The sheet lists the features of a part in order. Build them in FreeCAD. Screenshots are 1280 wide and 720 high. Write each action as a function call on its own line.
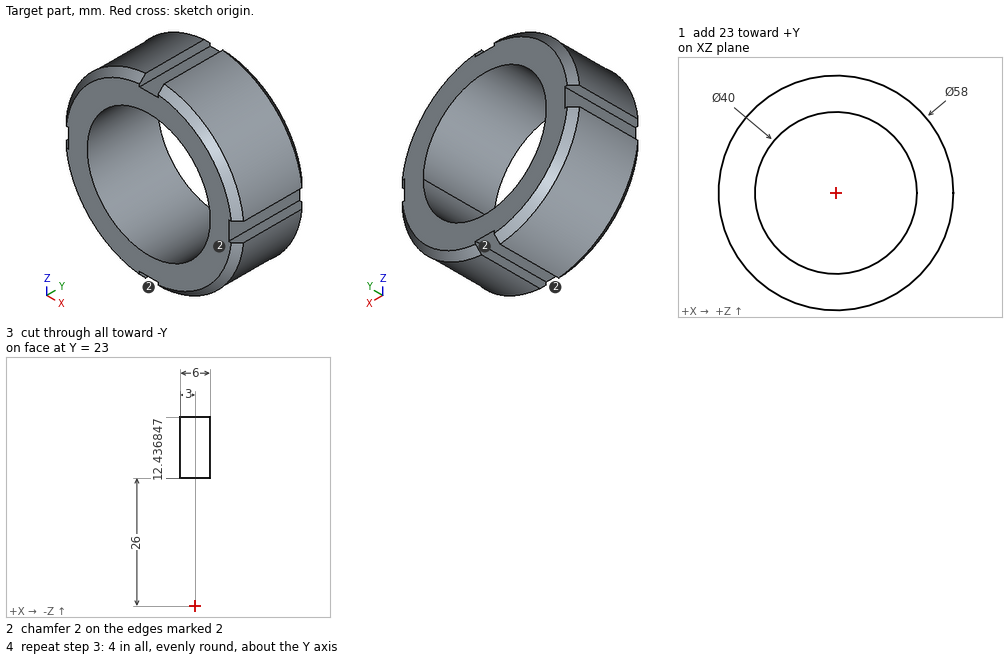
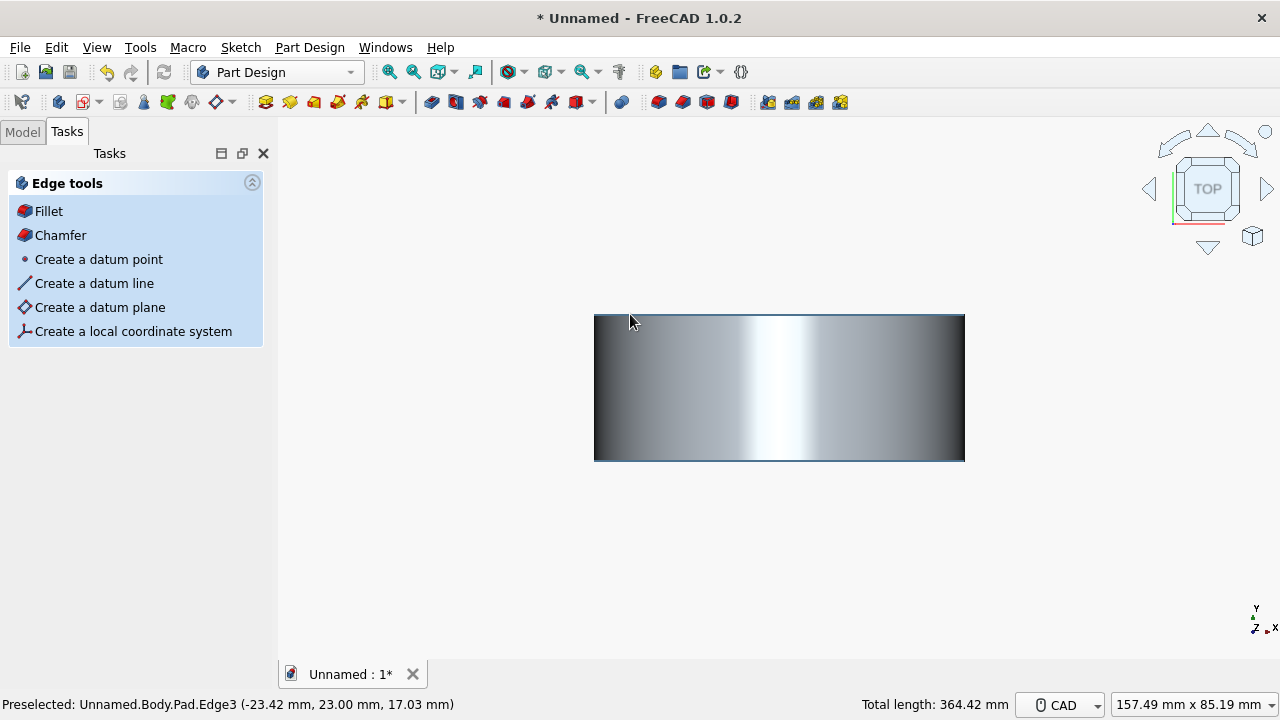
click(684, 102)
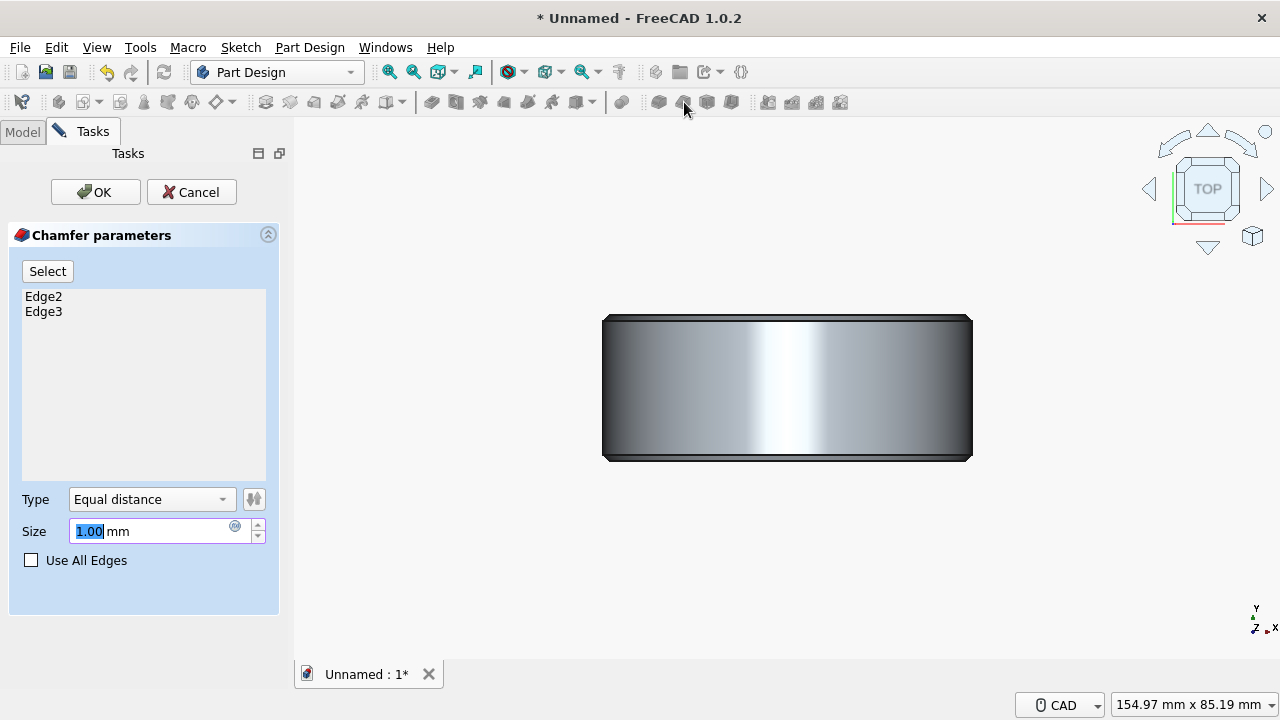
text(2)
key(Tab)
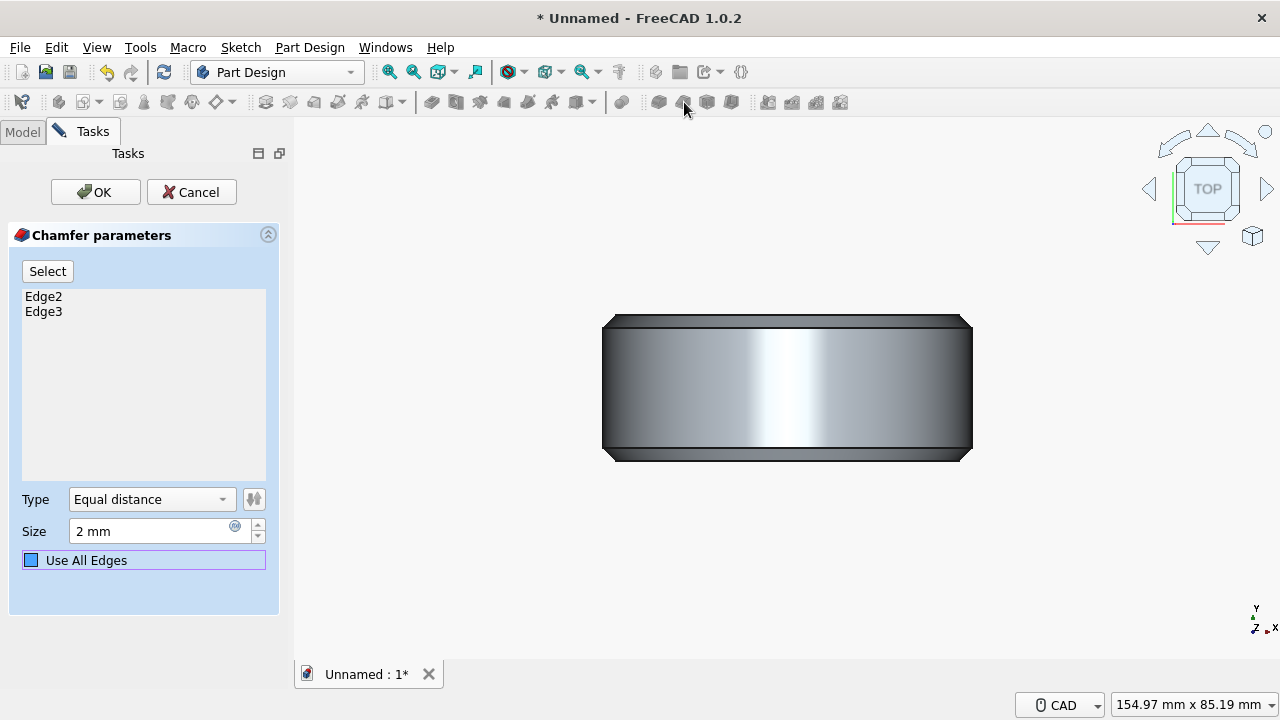
click(96, 192)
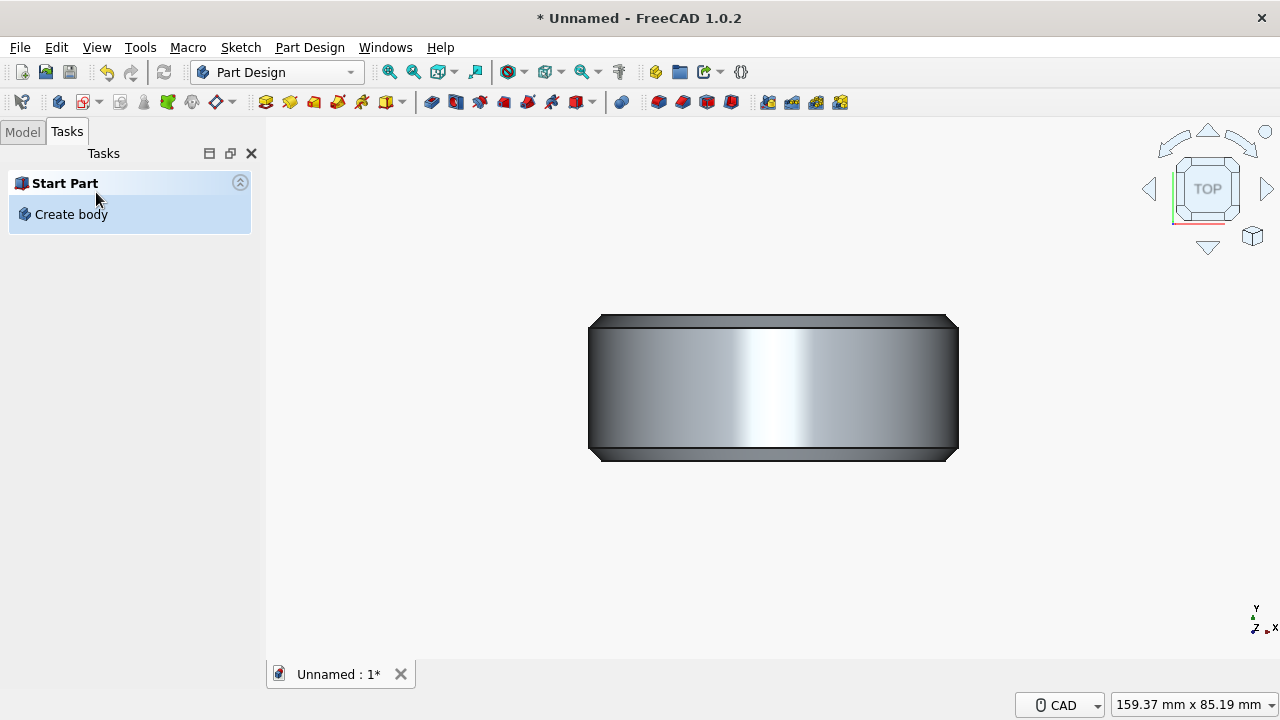
click(390, 72)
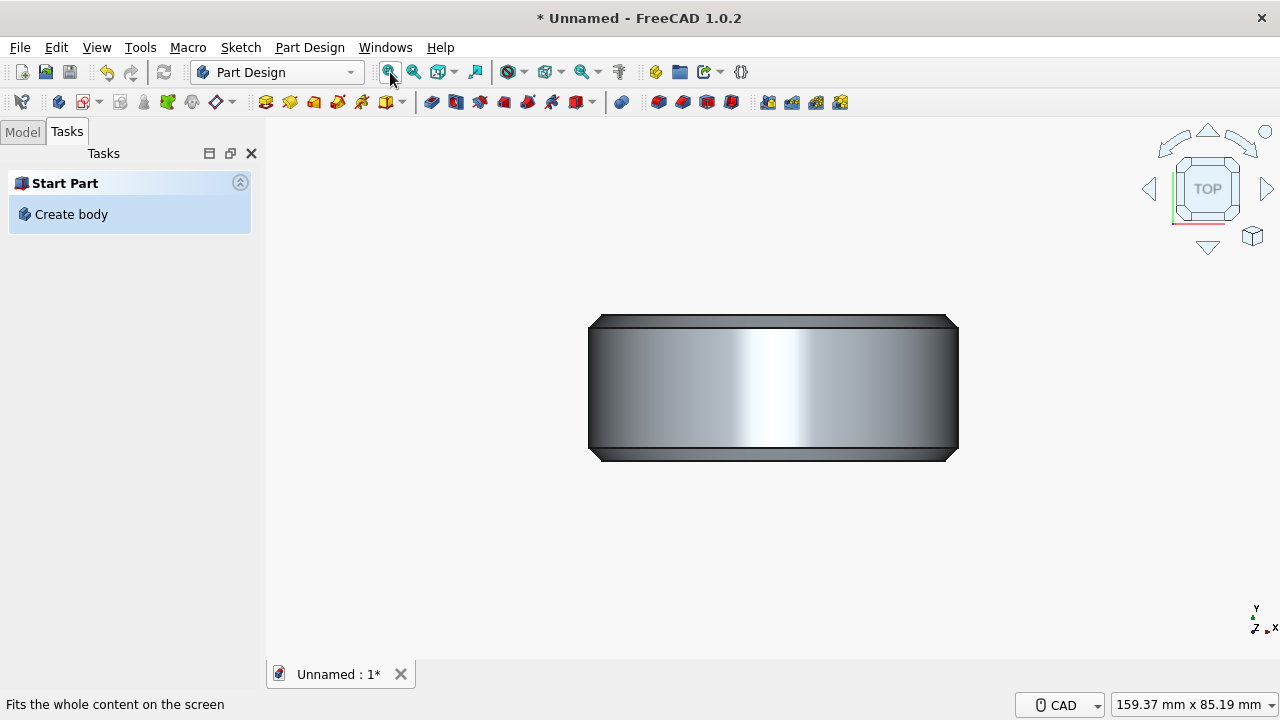
key(4)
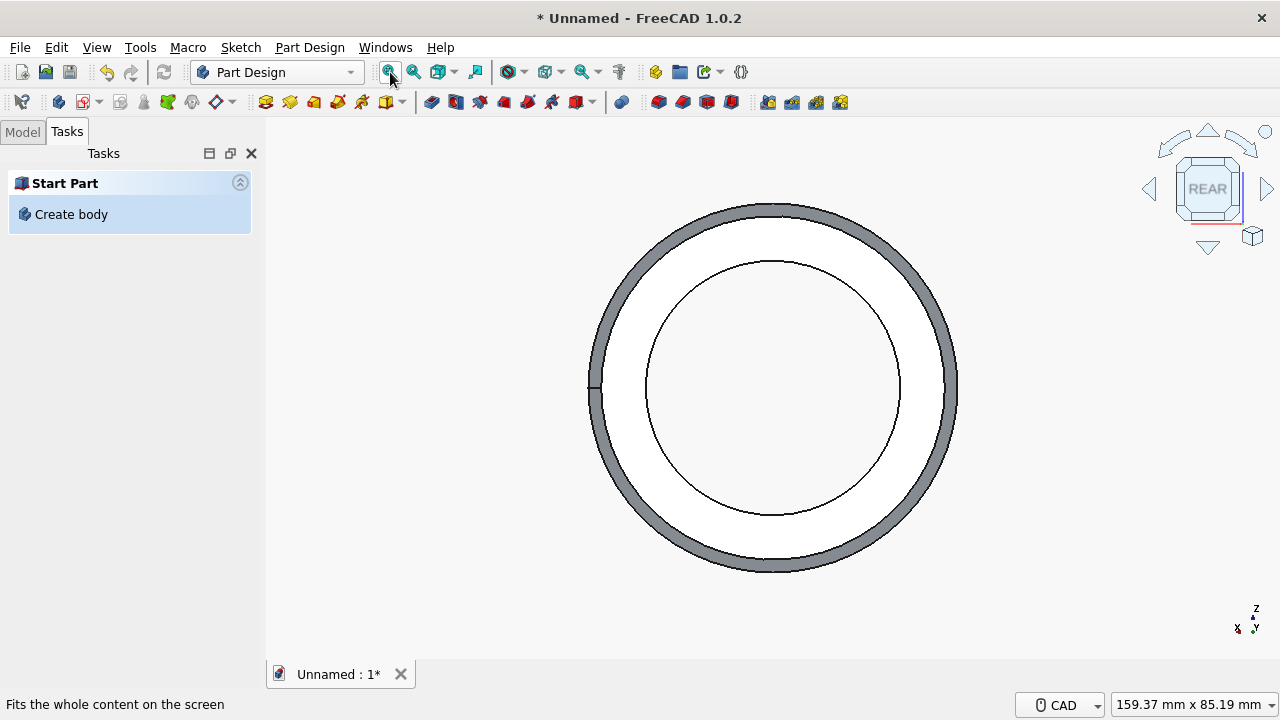
click(773, 240)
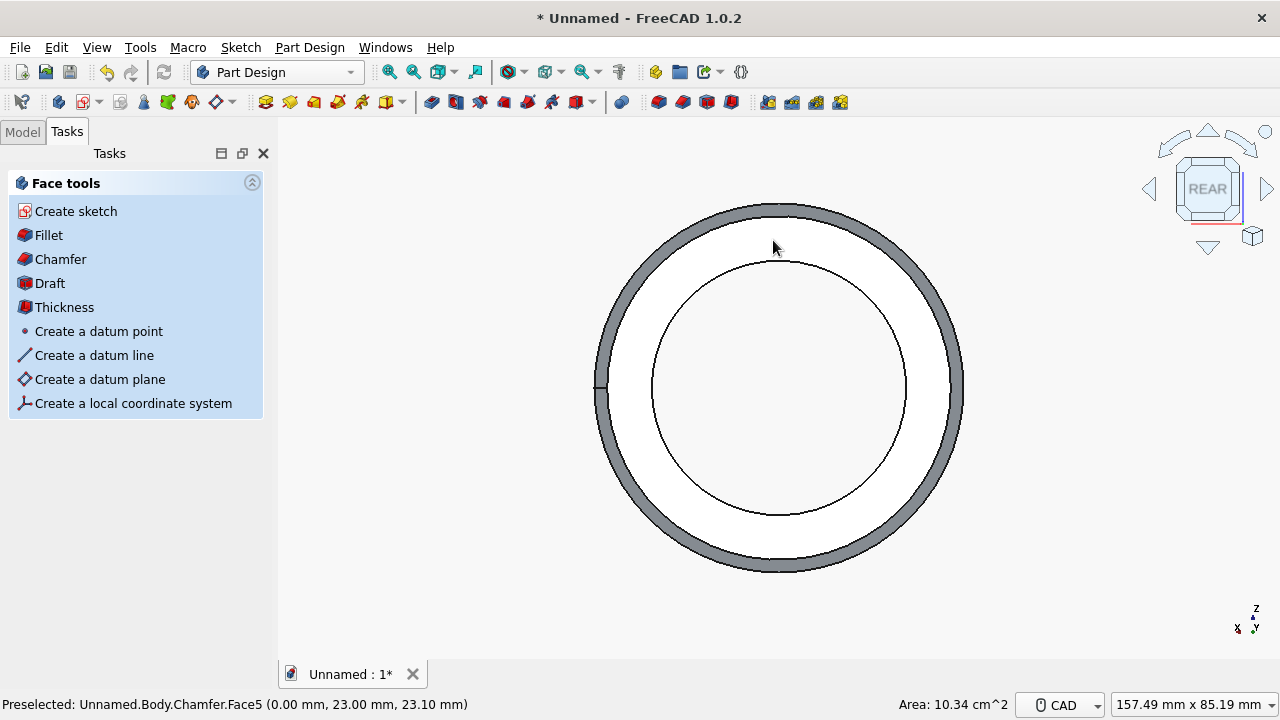
click(84, 102)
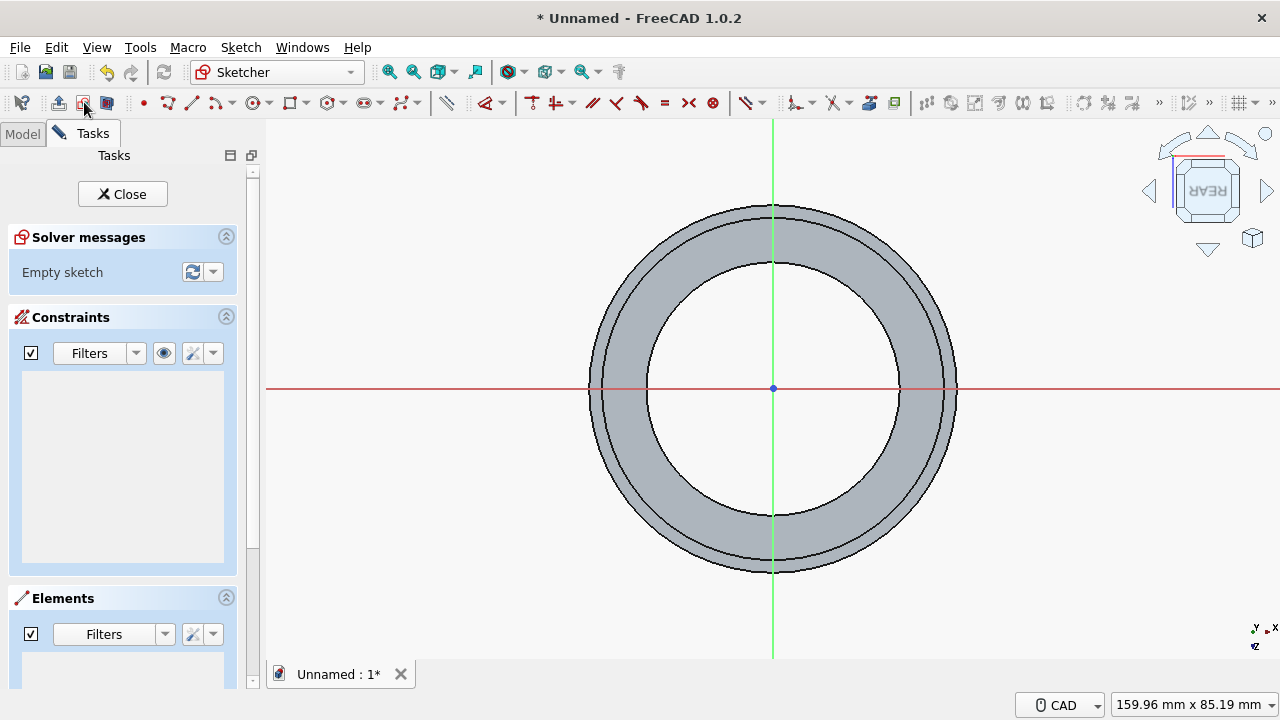
scroll(704, 389, down, 5)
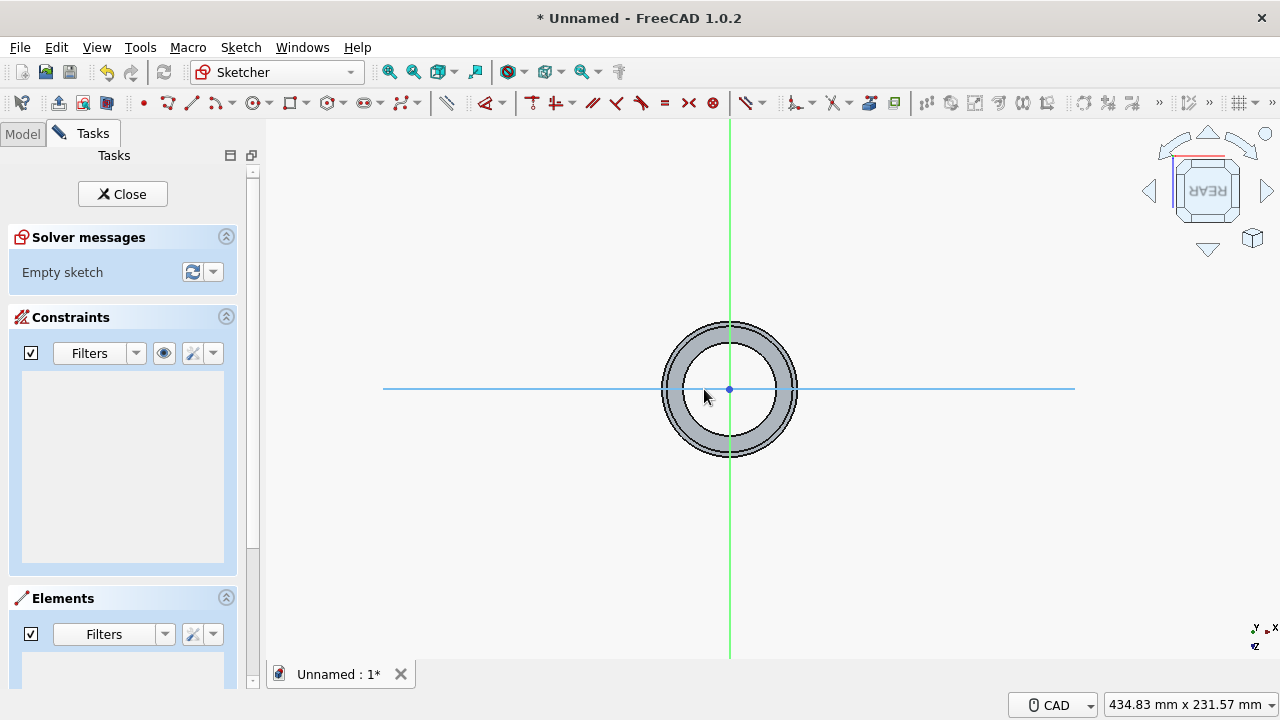
scroll(732, 307, up, 12)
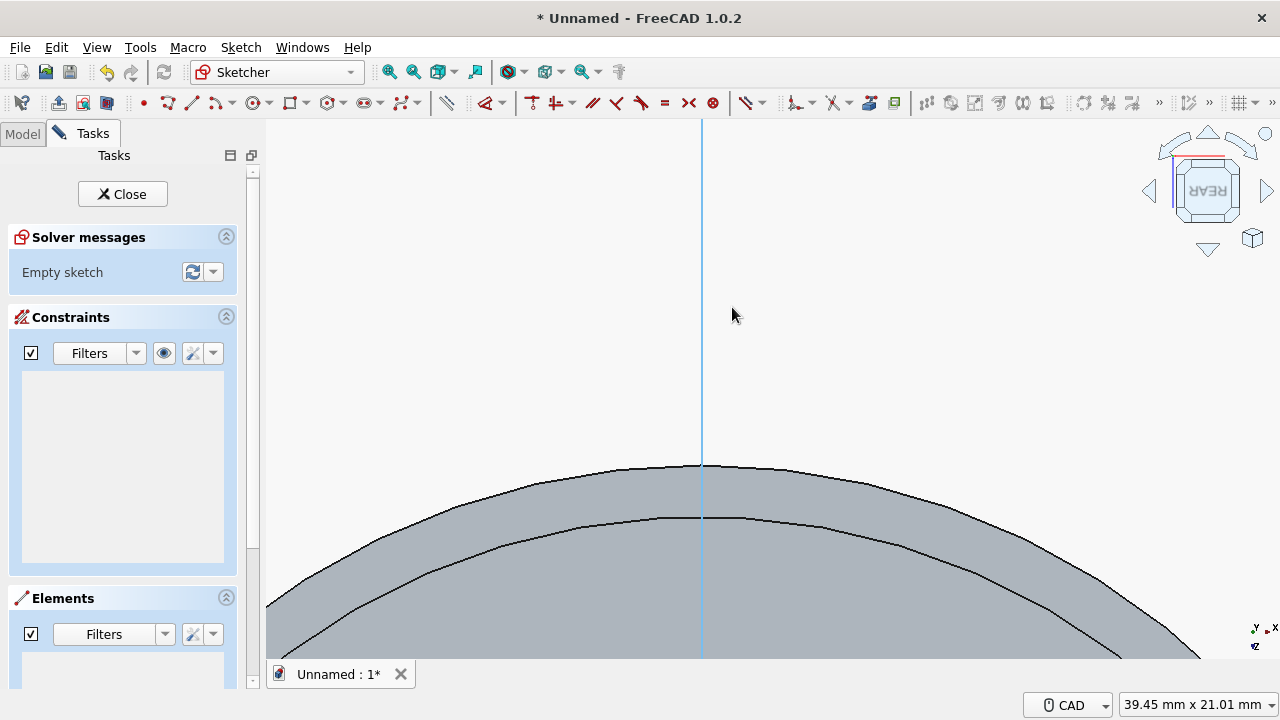
click(290, 104)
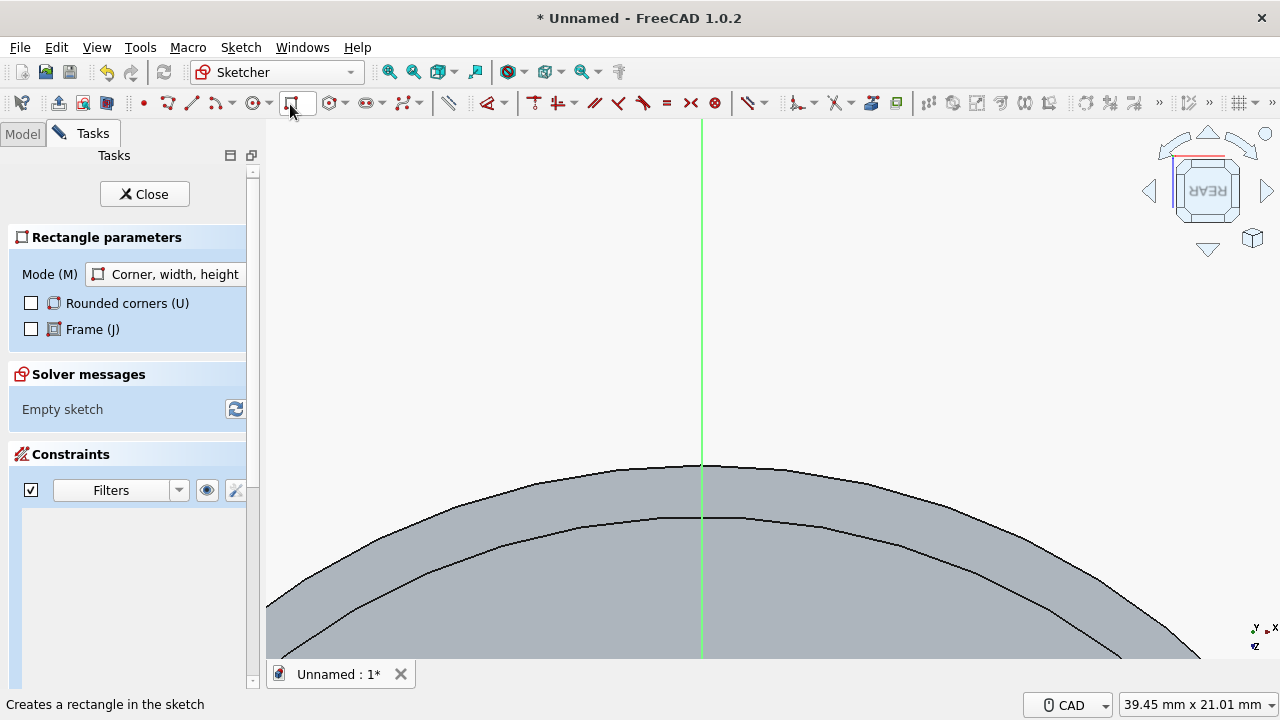
click(624, 223)
click(779, 543)
key(Escape)